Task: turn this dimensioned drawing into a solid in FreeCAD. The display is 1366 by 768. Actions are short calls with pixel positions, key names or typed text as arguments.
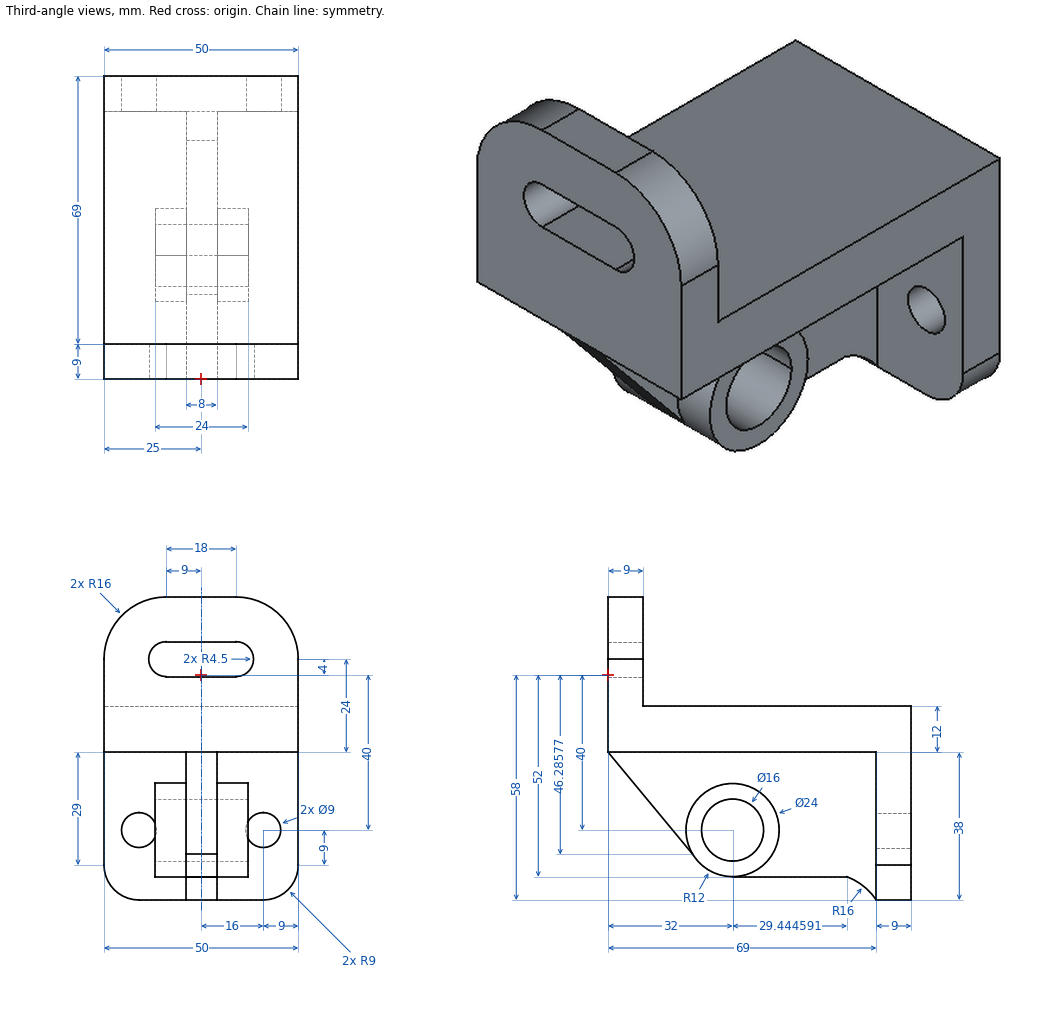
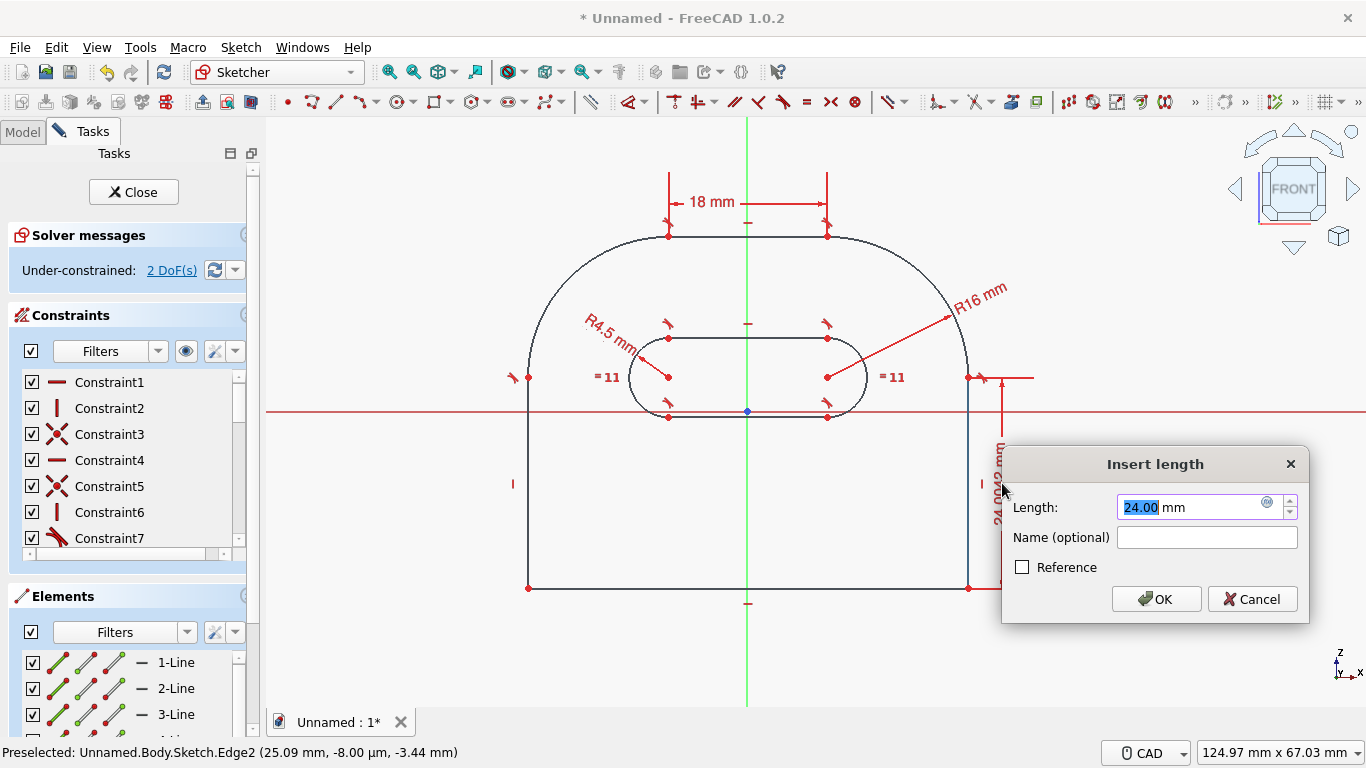
text(24)
key(Return)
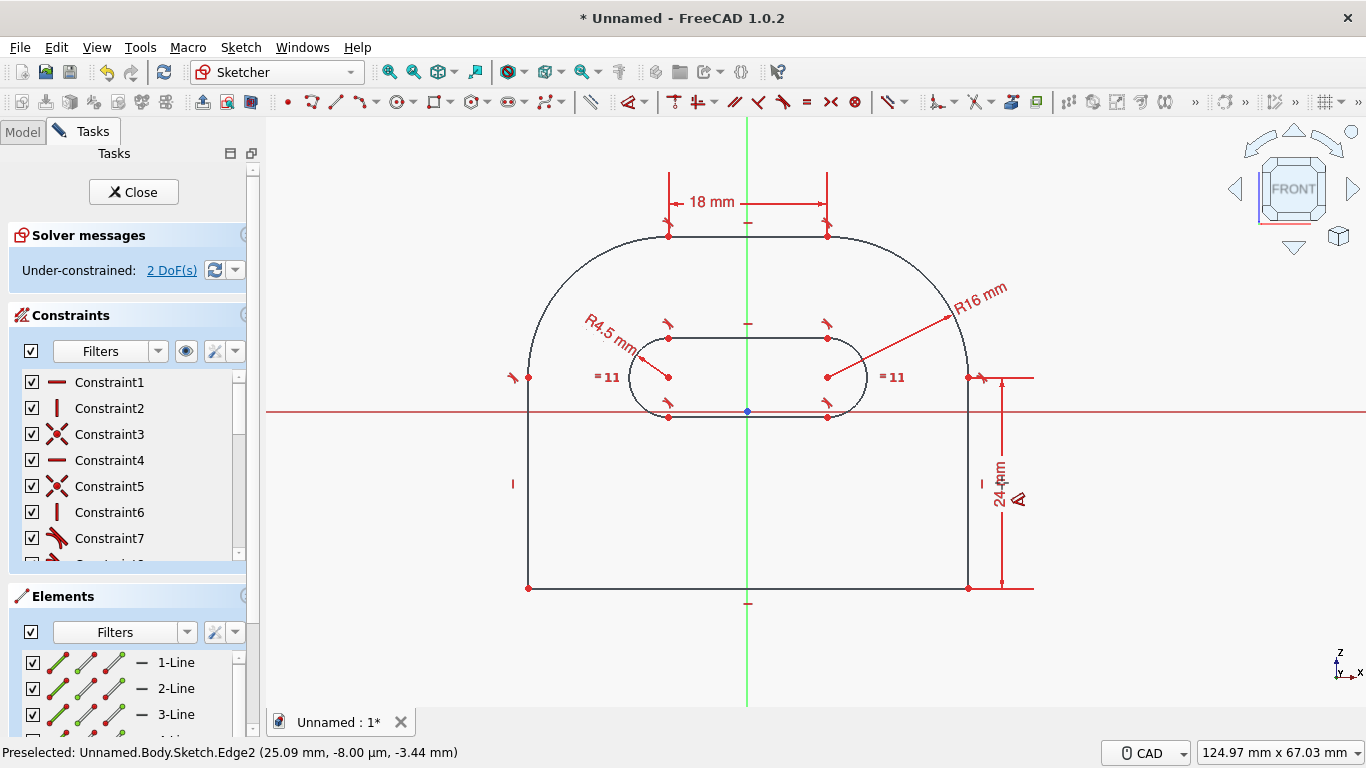
click(669, 237)
click(708, 446)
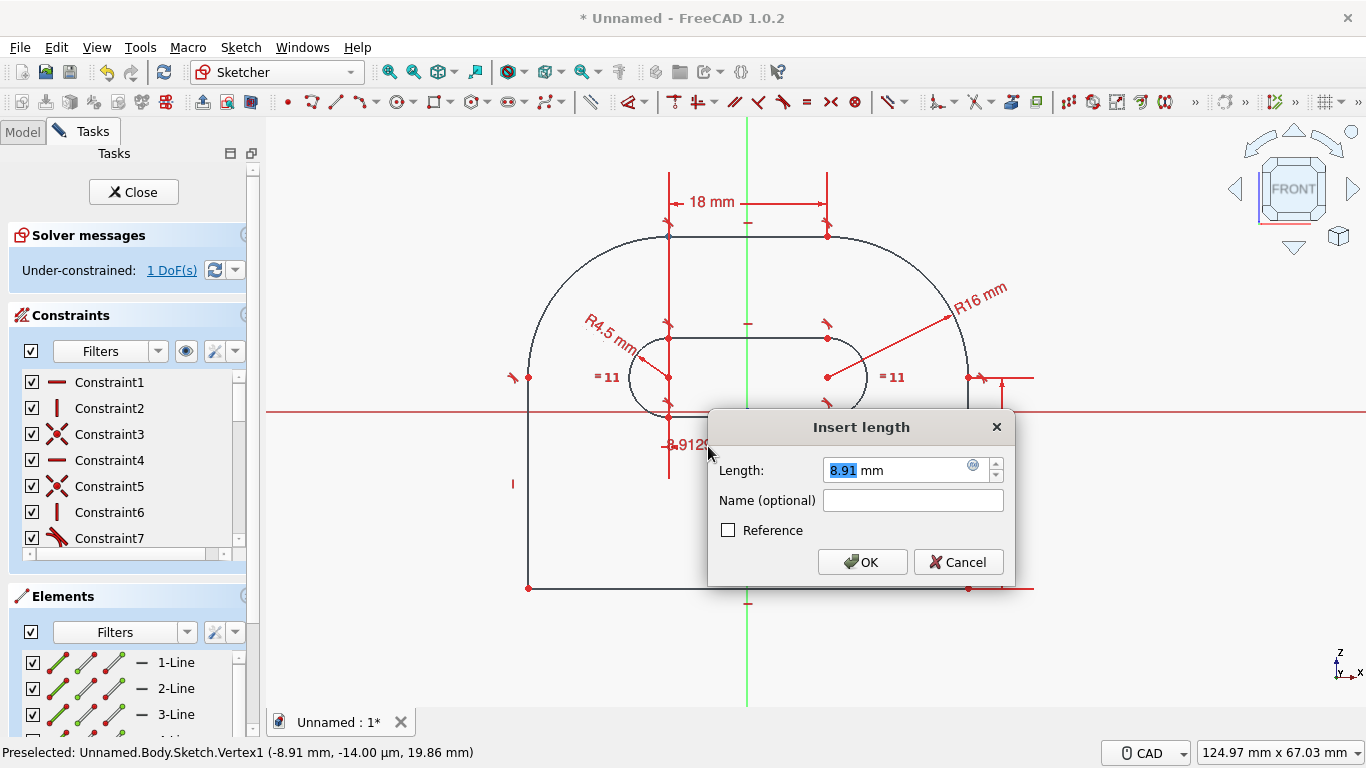
text(9)
key(Return)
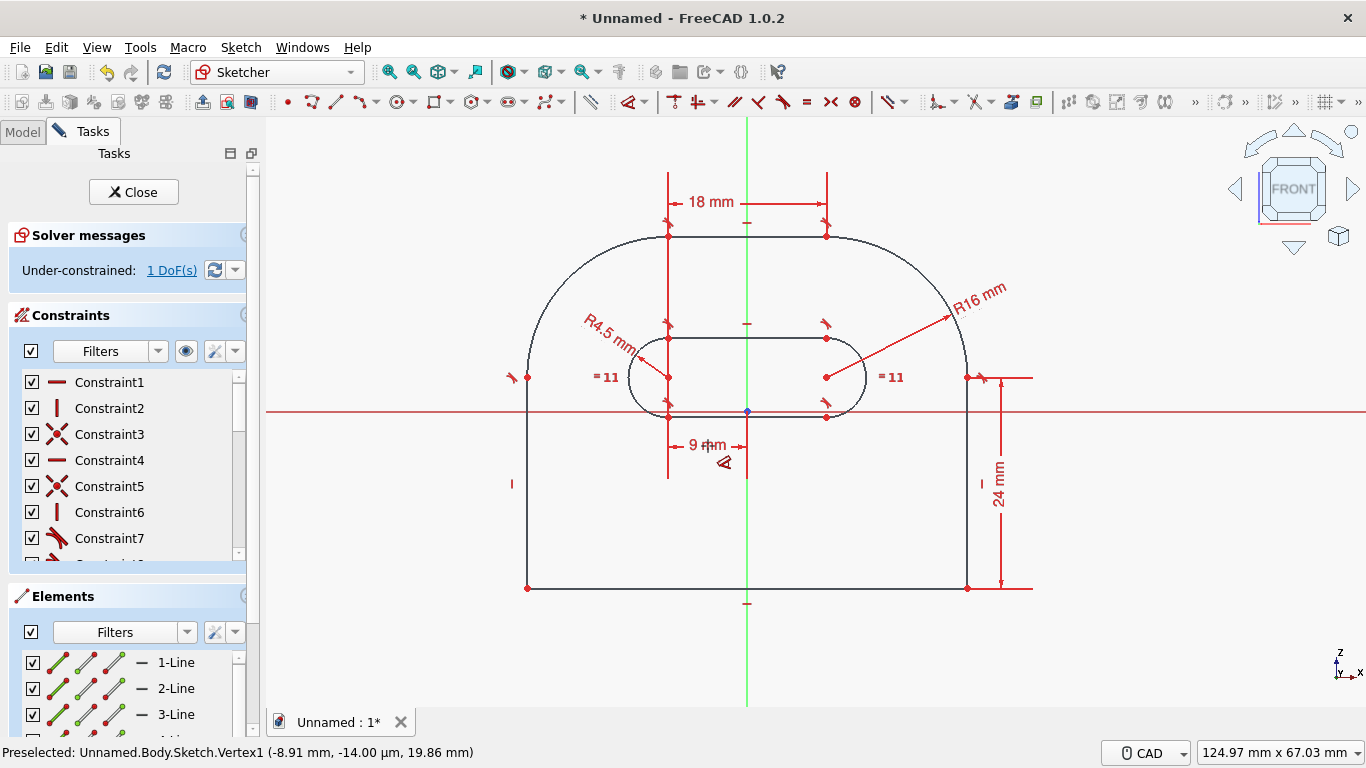
click(967, 378)
click(1001, 395)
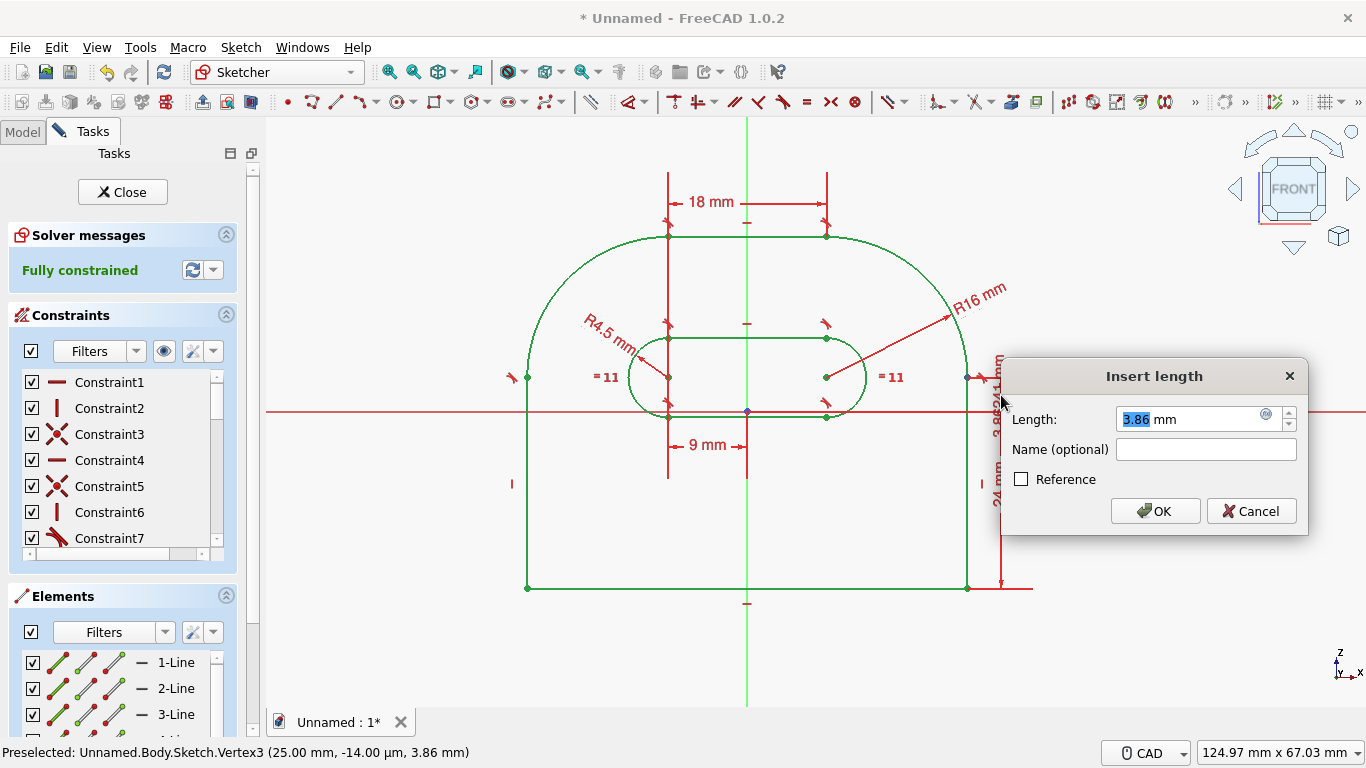
text(4)
key(Return)
key(Escape)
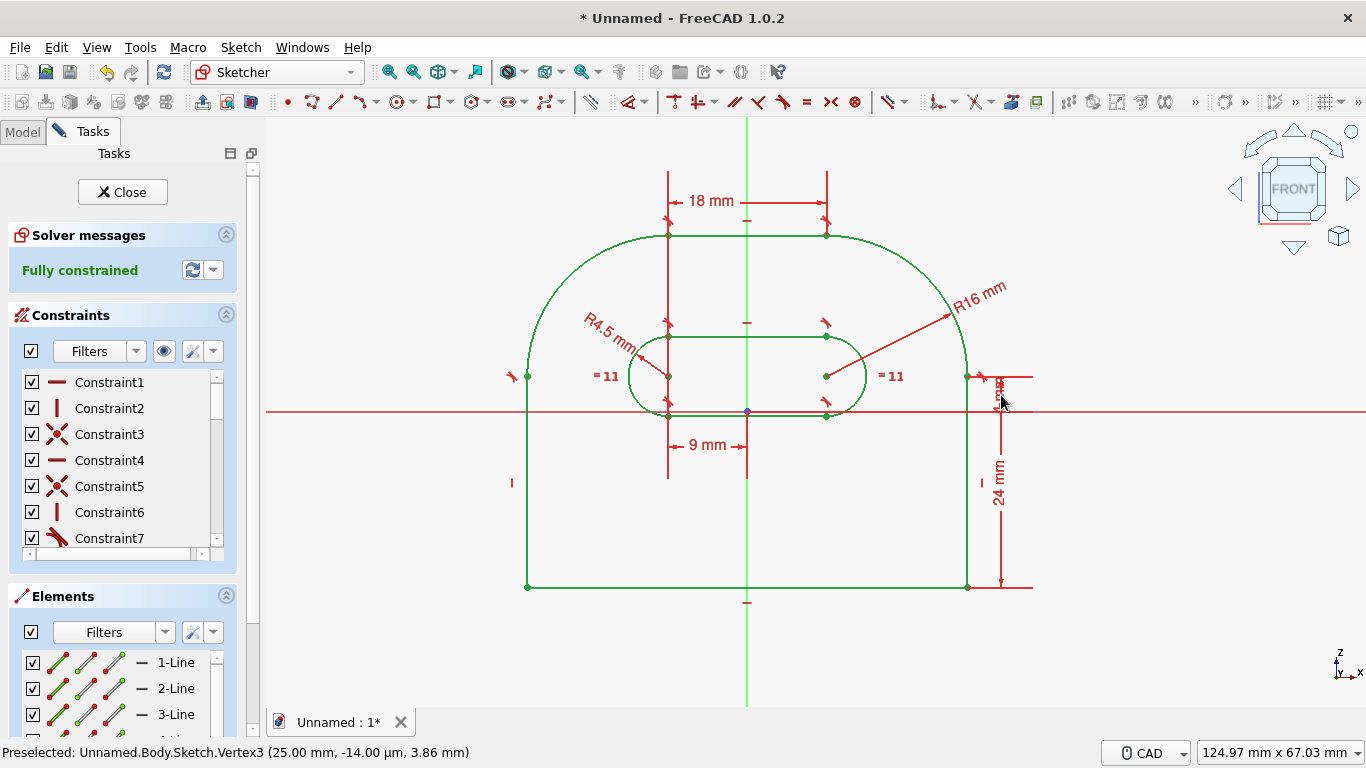
click(123, 192)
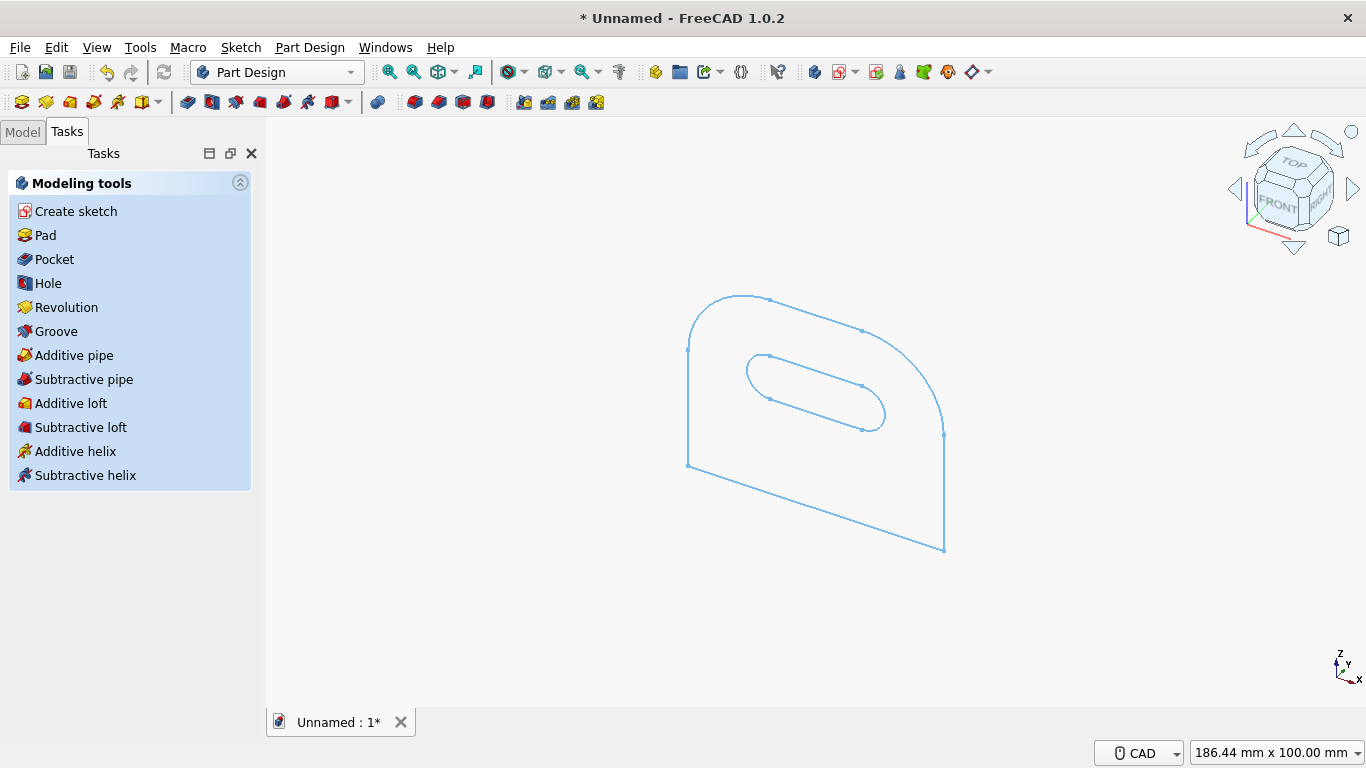
click(22, 102)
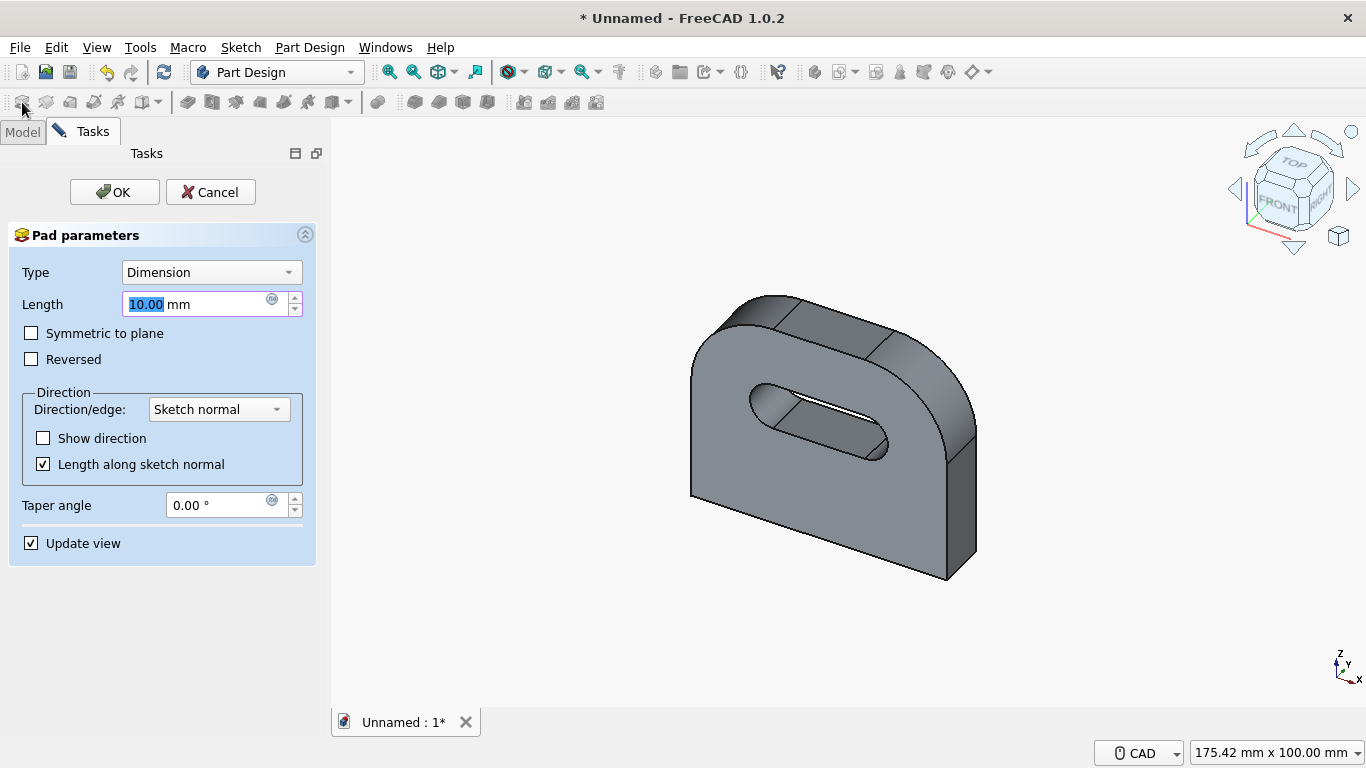
text(9)
key(Tab)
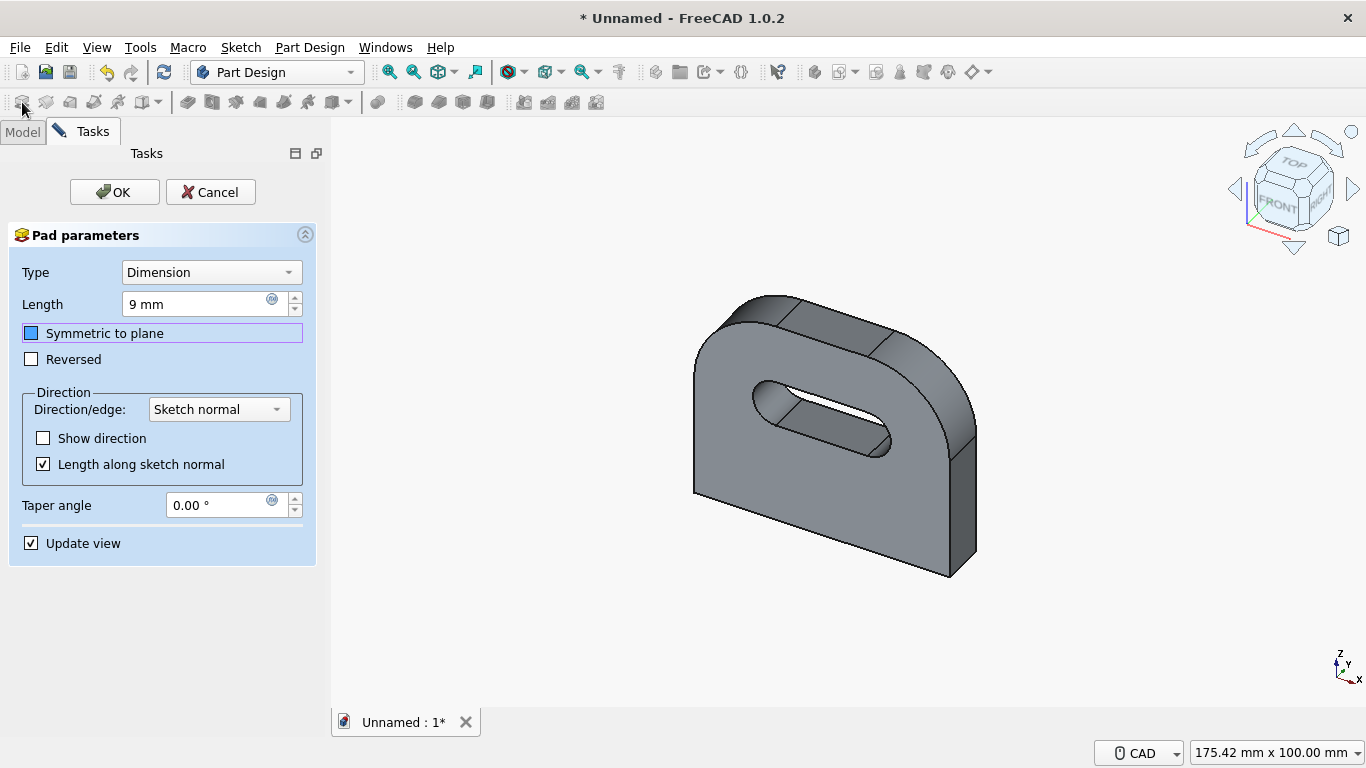
click(30, 359)